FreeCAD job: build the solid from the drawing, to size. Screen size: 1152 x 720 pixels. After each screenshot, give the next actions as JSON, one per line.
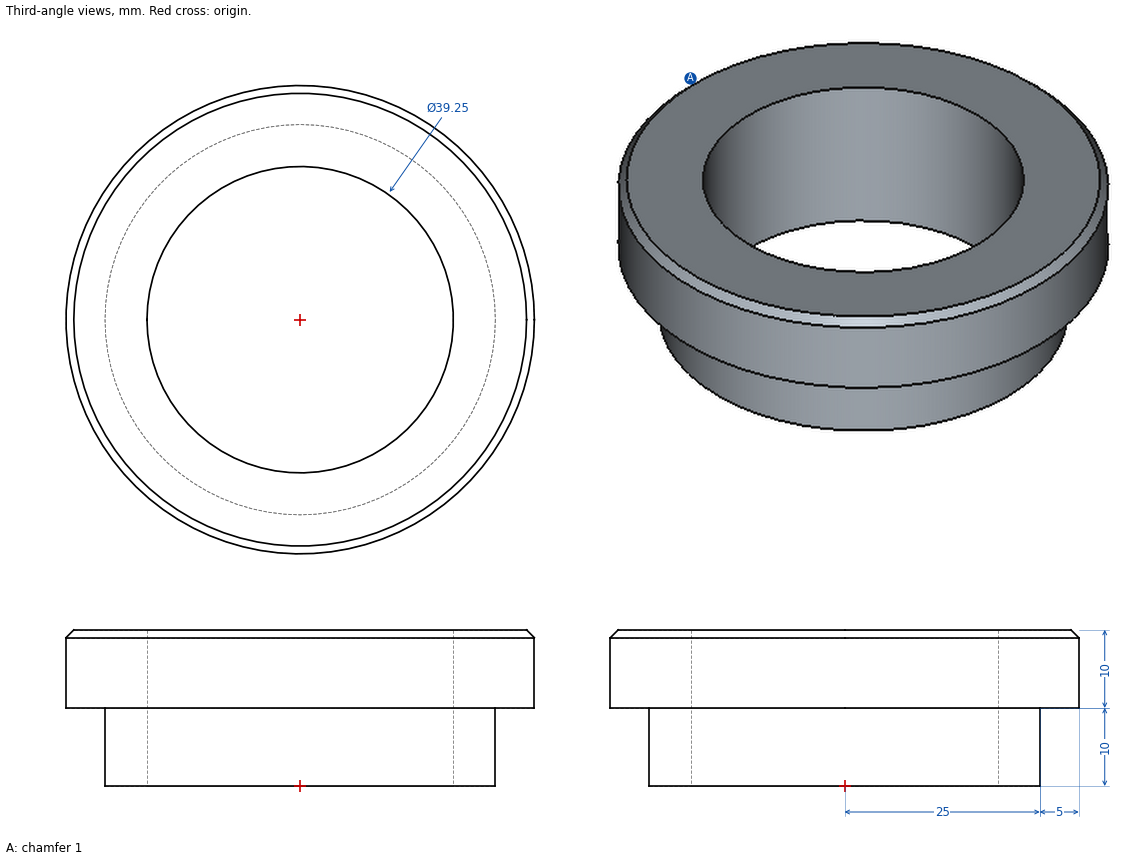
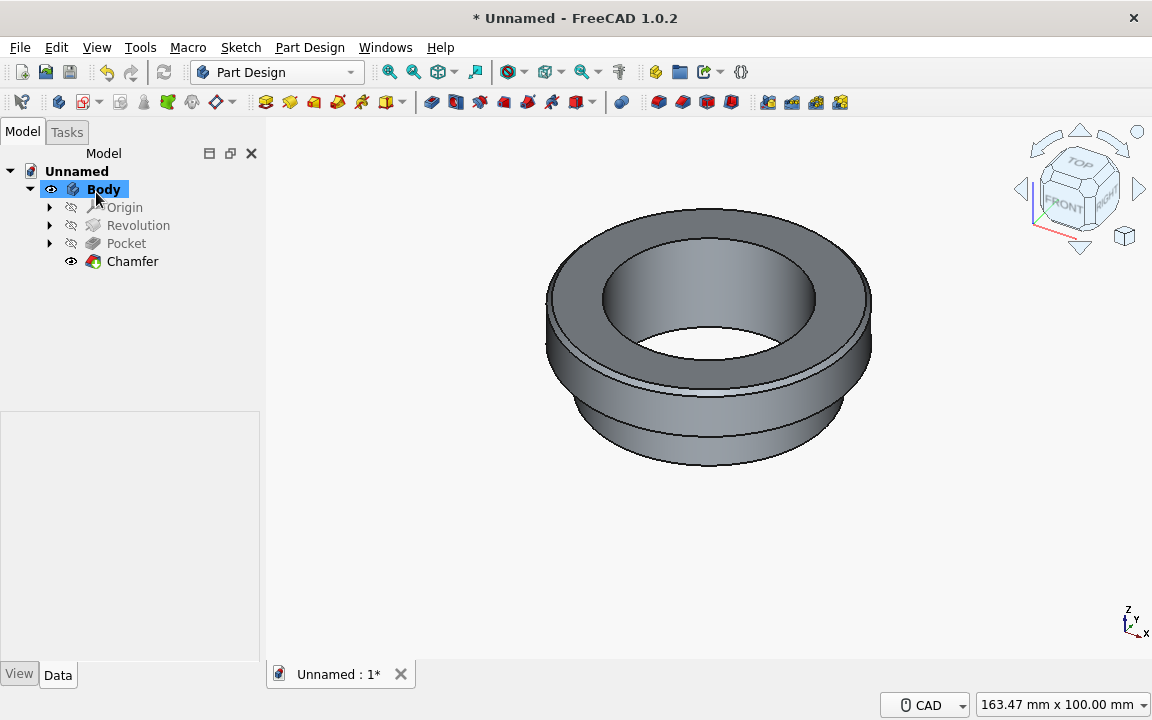
{"action": "key", "text": "0"}